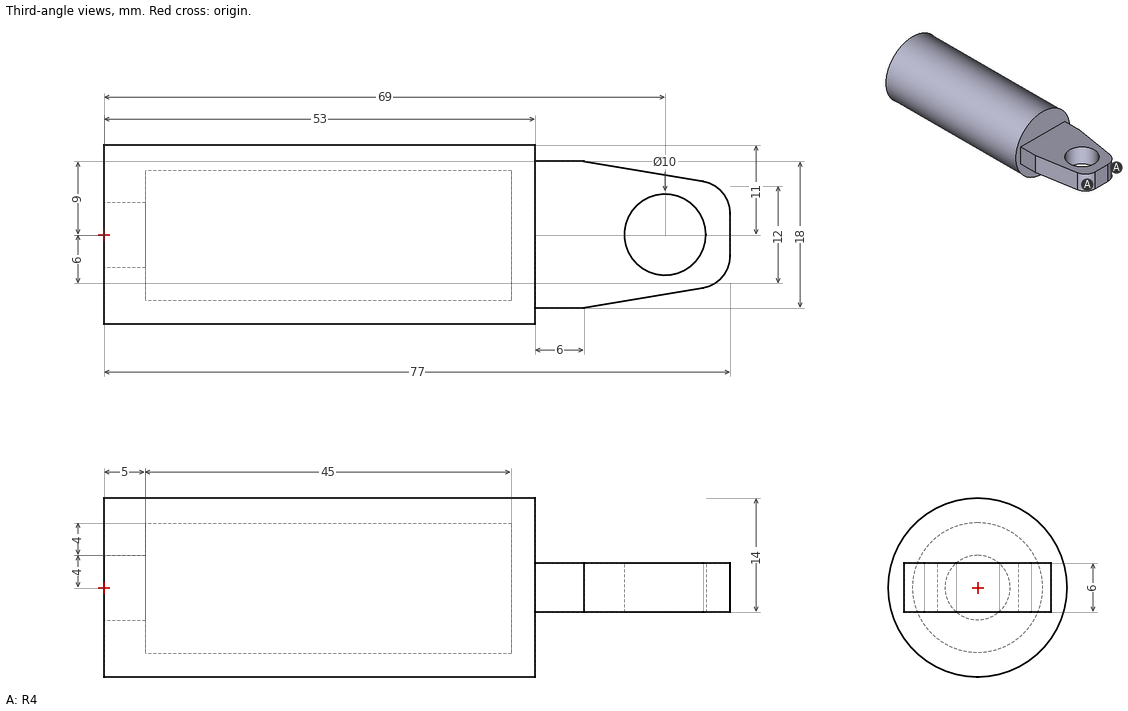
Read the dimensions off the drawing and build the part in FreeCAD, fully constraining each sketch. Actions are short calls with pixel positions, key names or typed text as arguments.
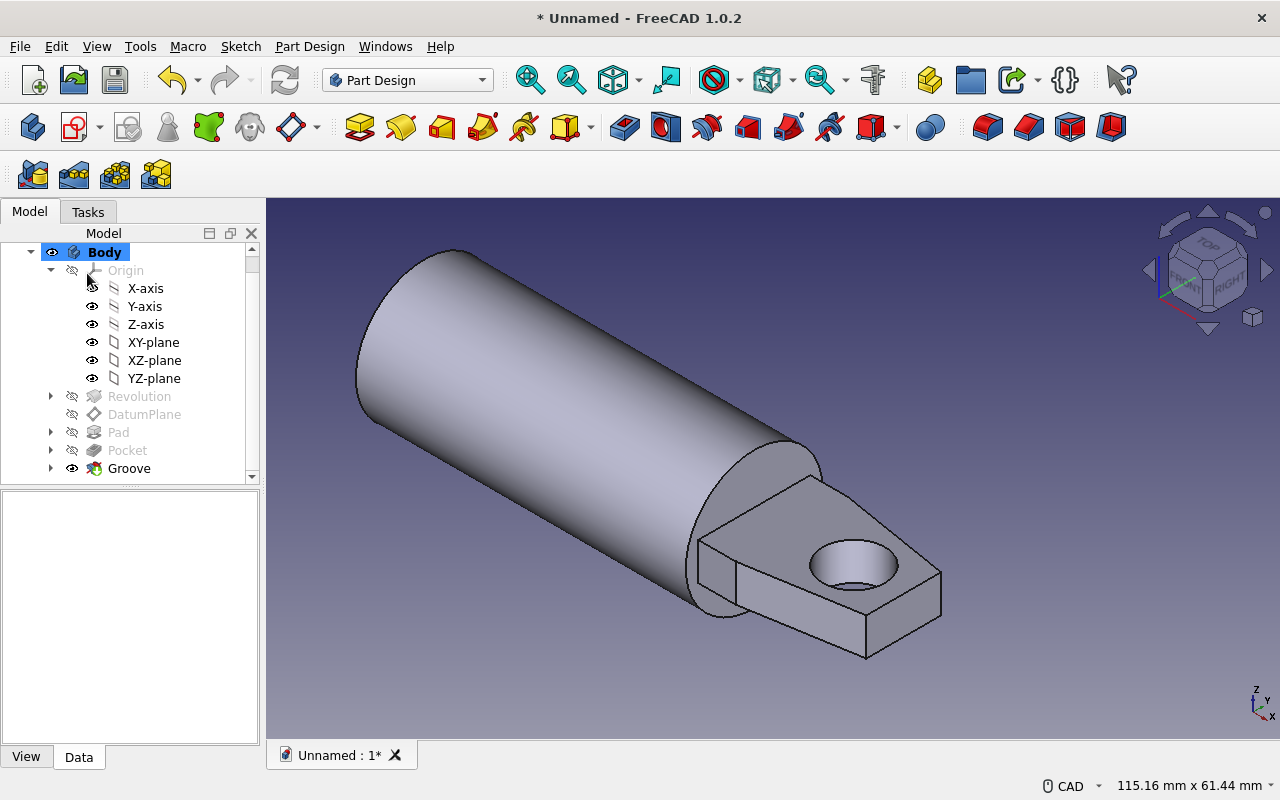
click(866, 636)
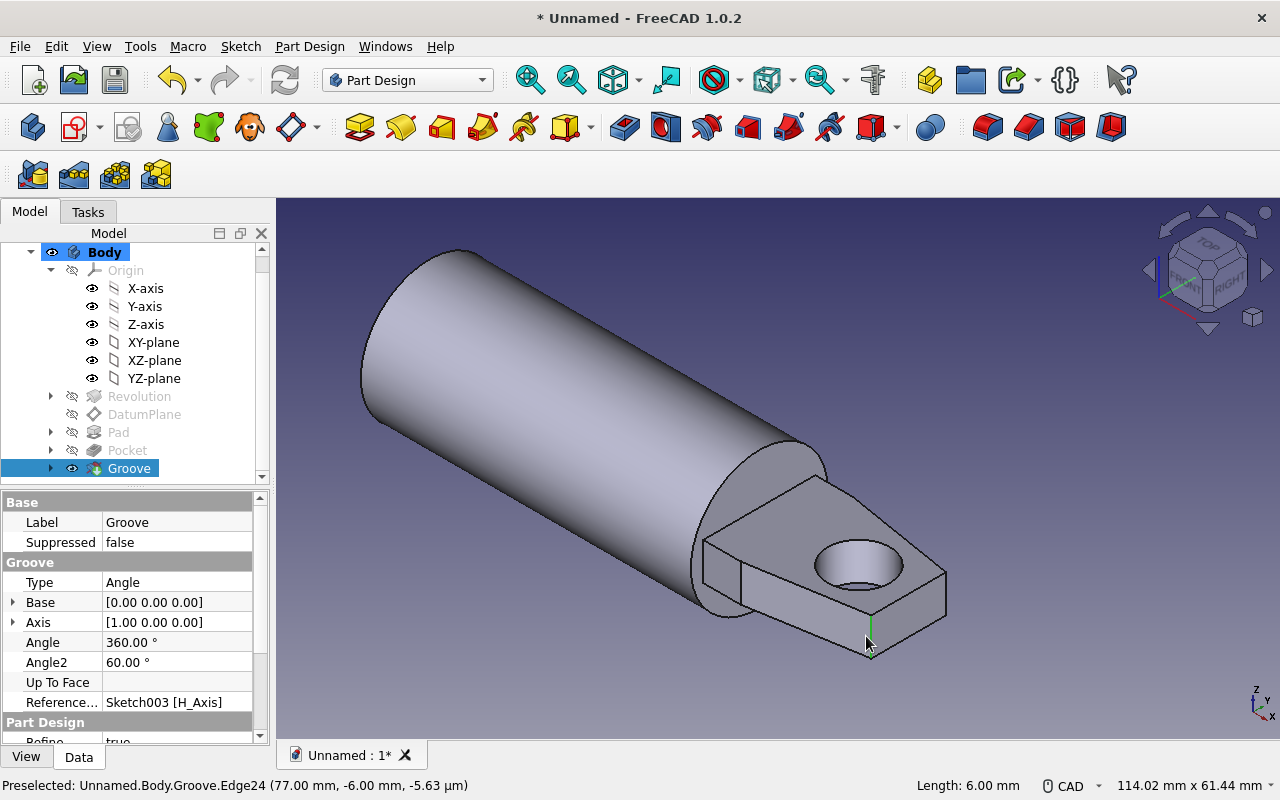
key(2)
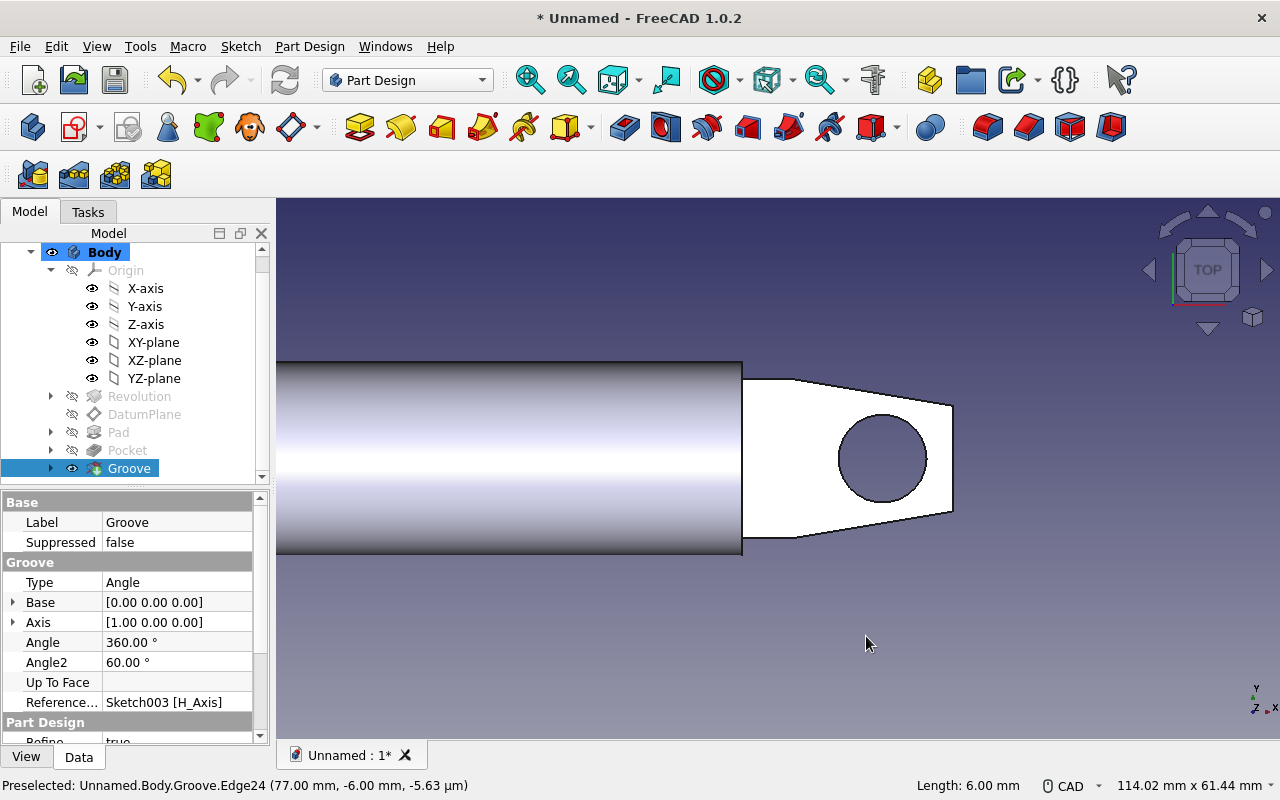
key(v)
key(f)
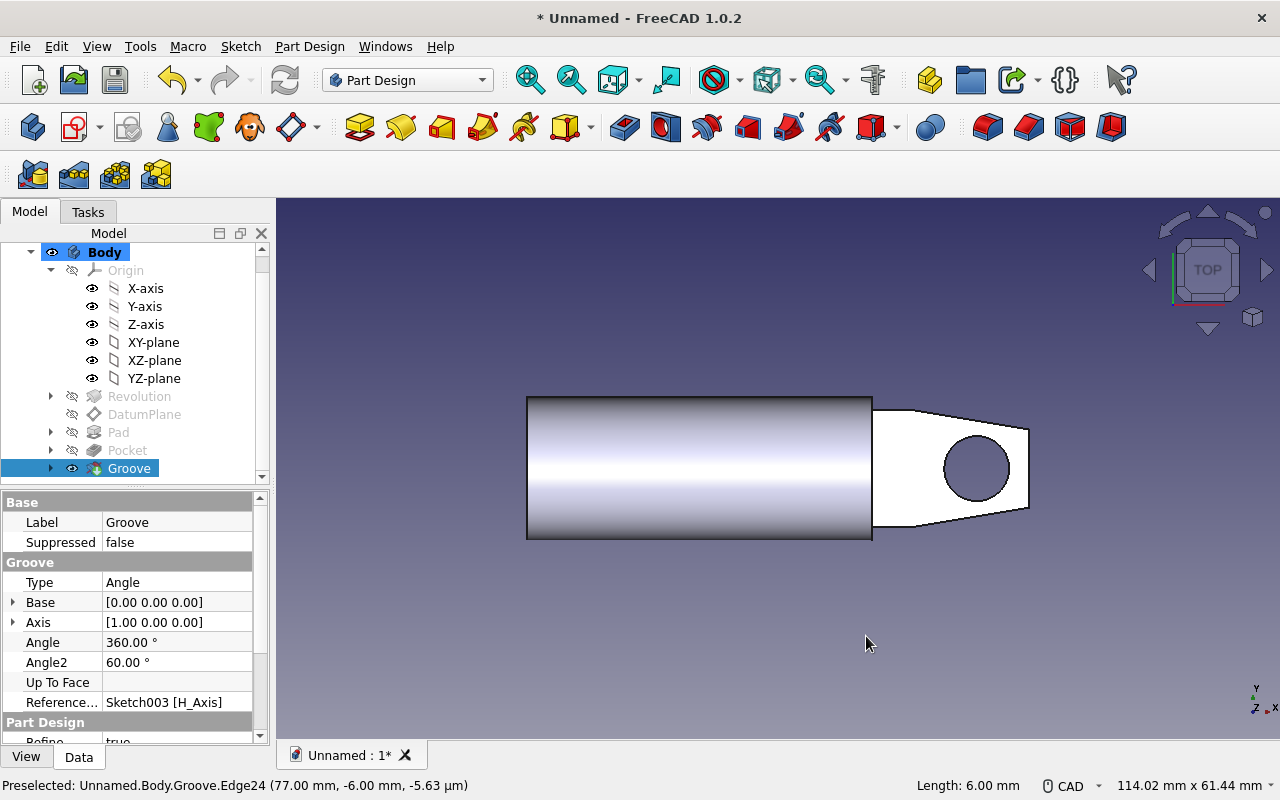
key(1)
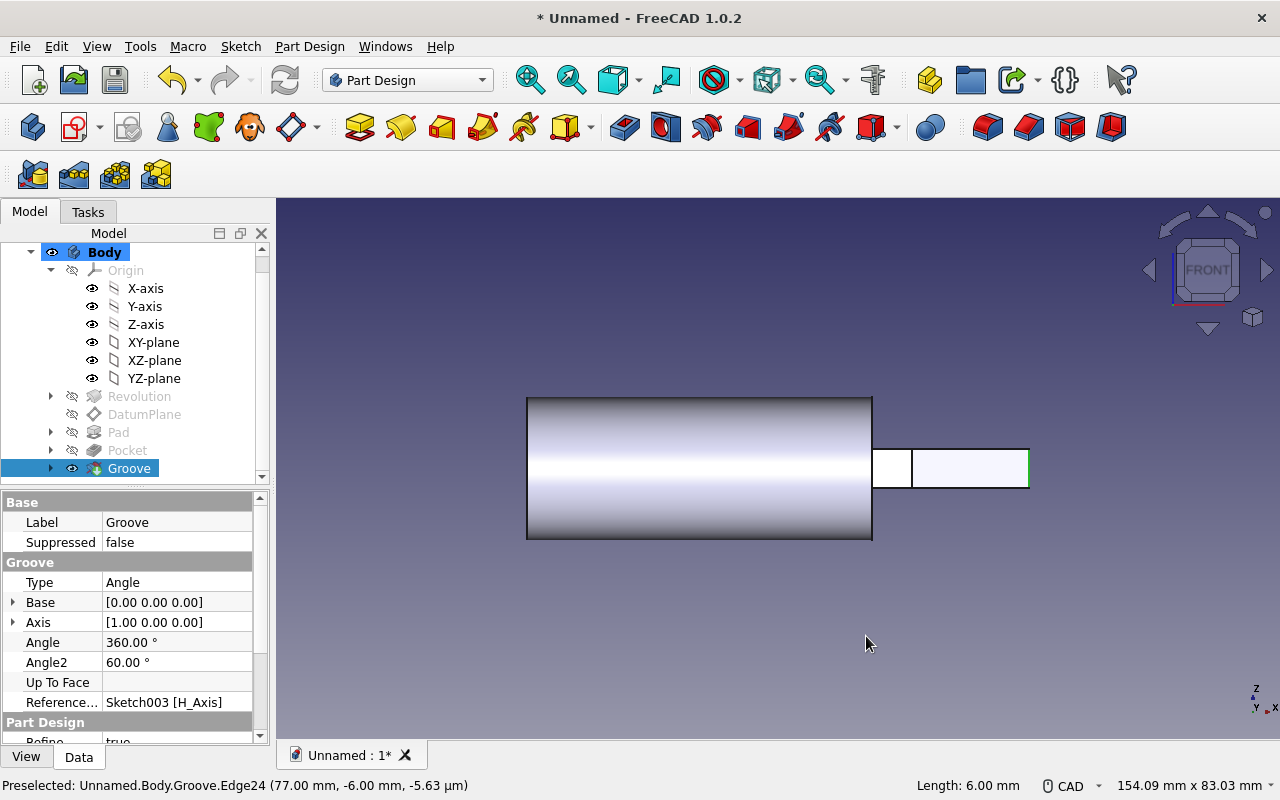
key(3)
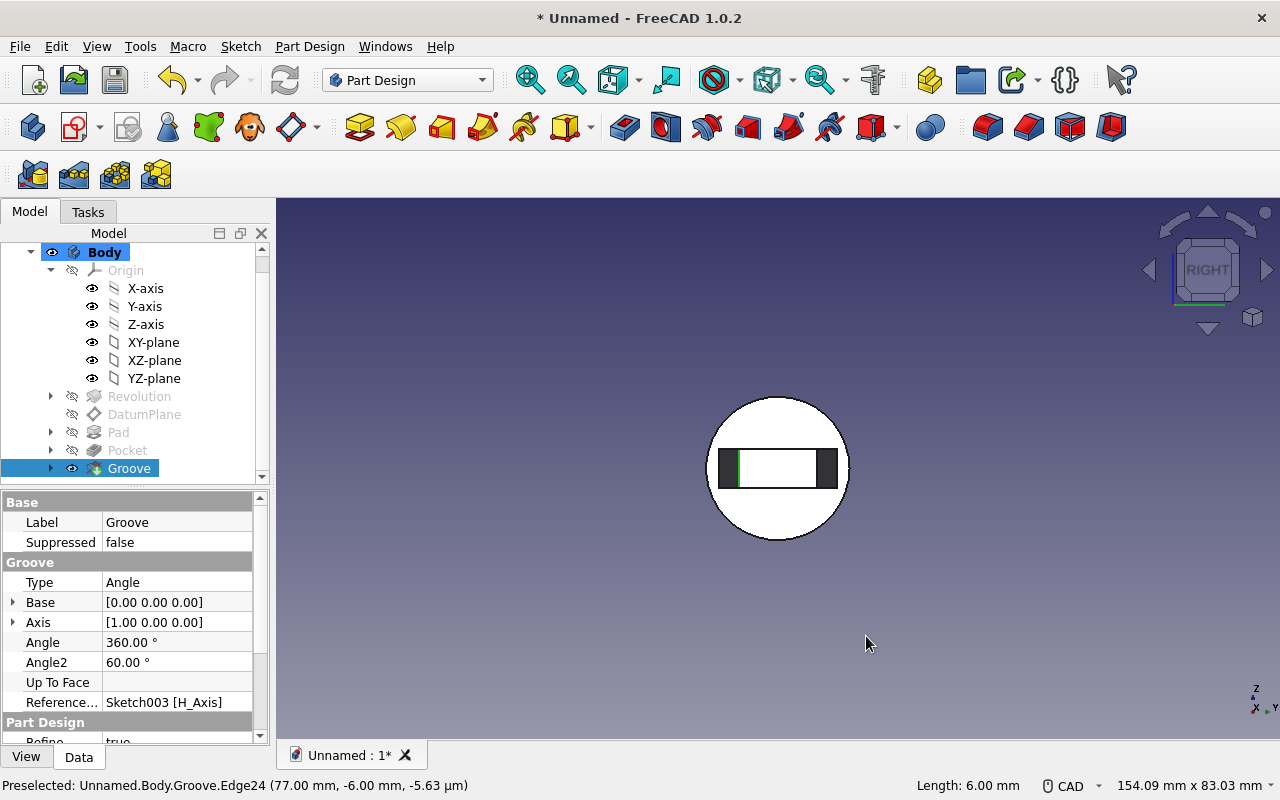
key(v)
key(f)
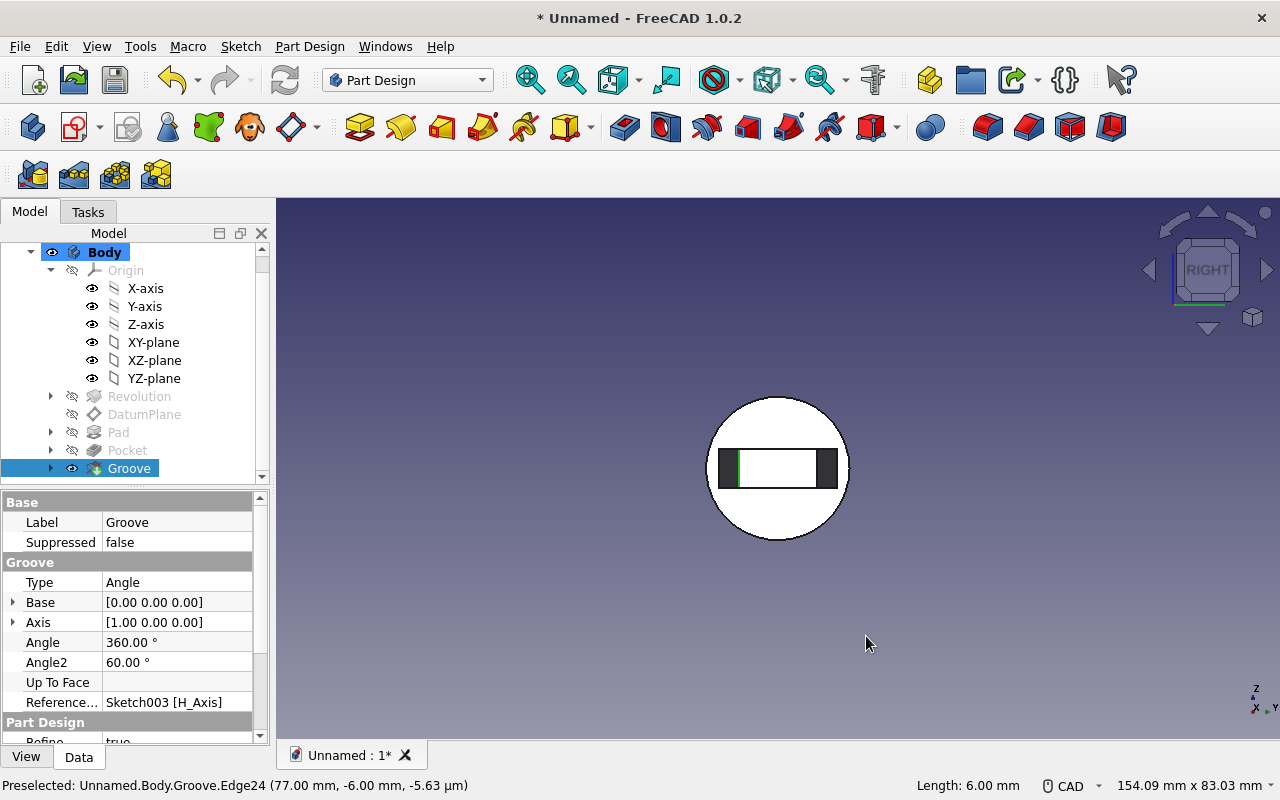
click(817, 467, ctrl)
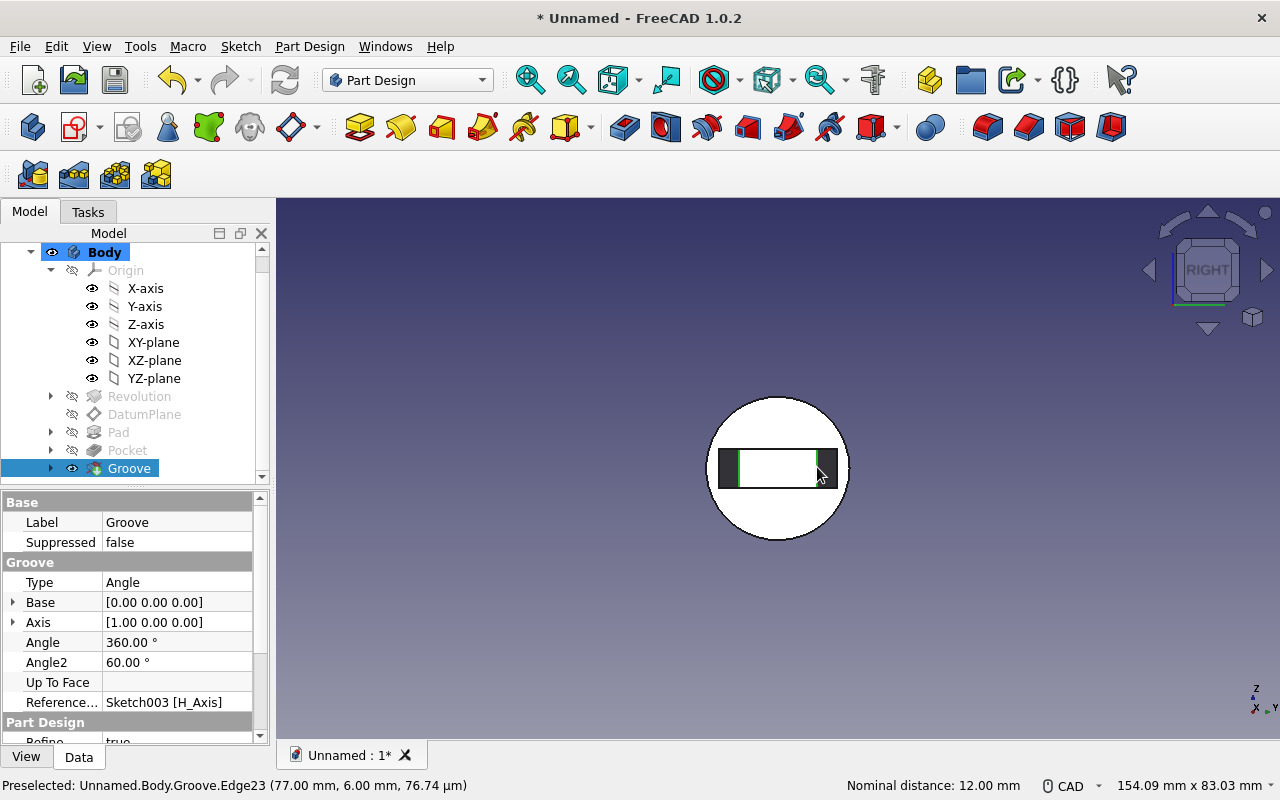
click(988, 128)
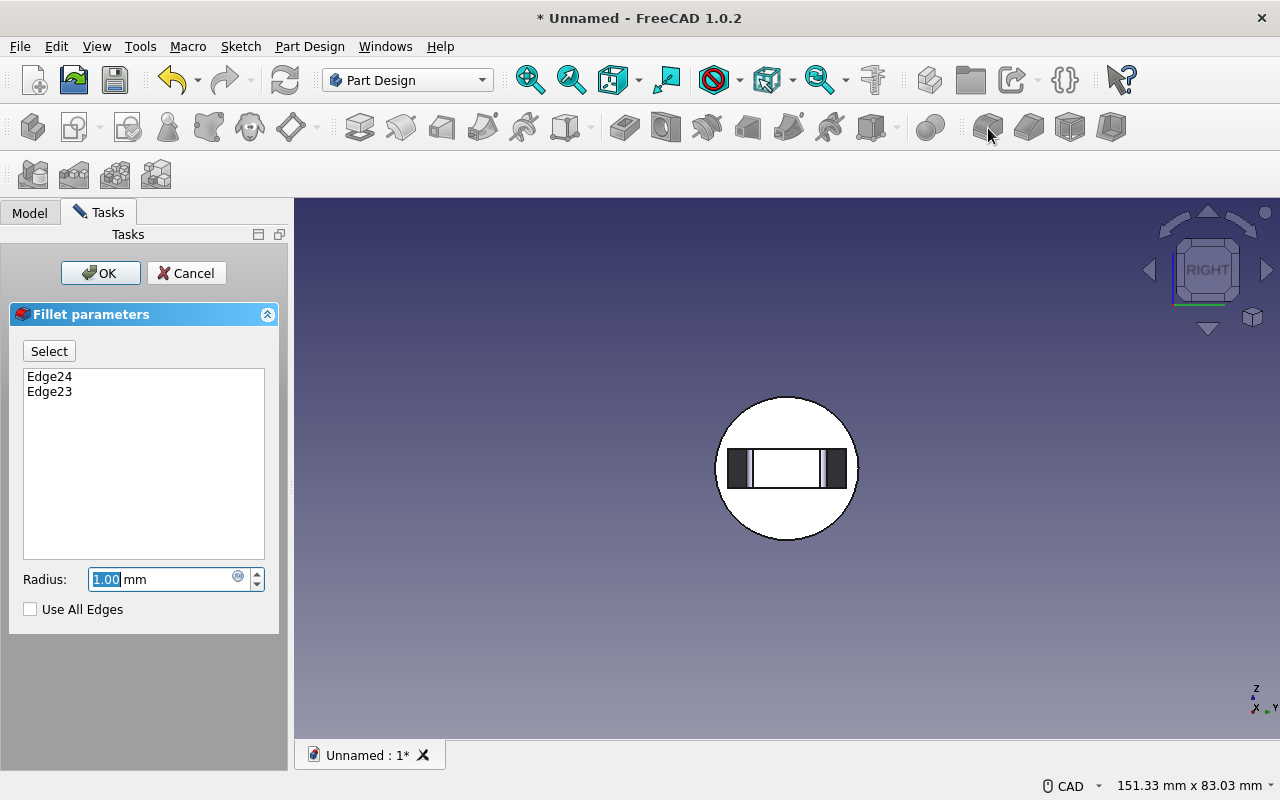
text(4)
key(Tab)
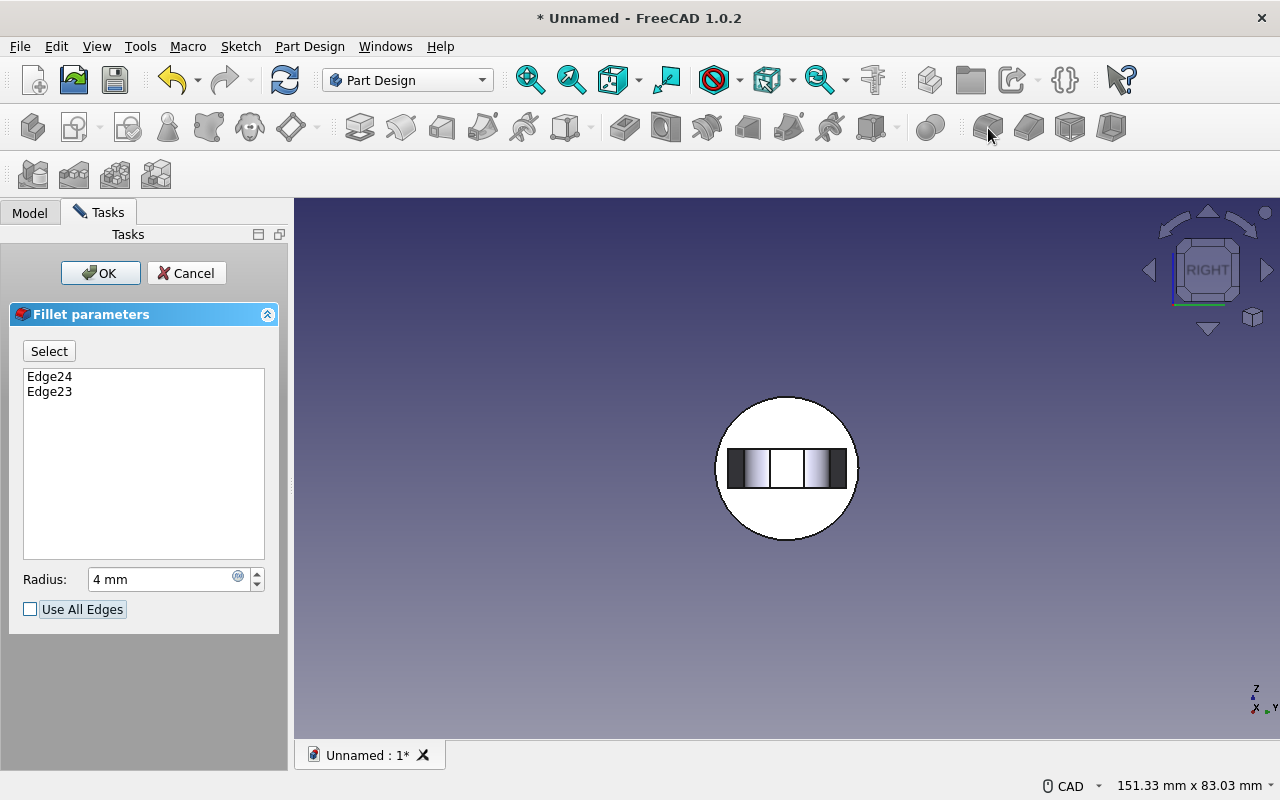
click(101, 273)